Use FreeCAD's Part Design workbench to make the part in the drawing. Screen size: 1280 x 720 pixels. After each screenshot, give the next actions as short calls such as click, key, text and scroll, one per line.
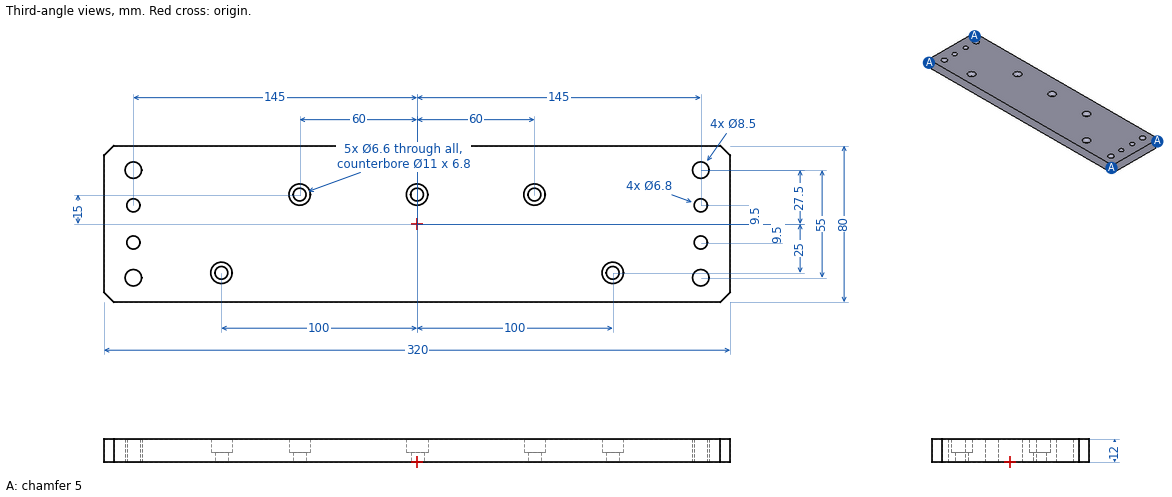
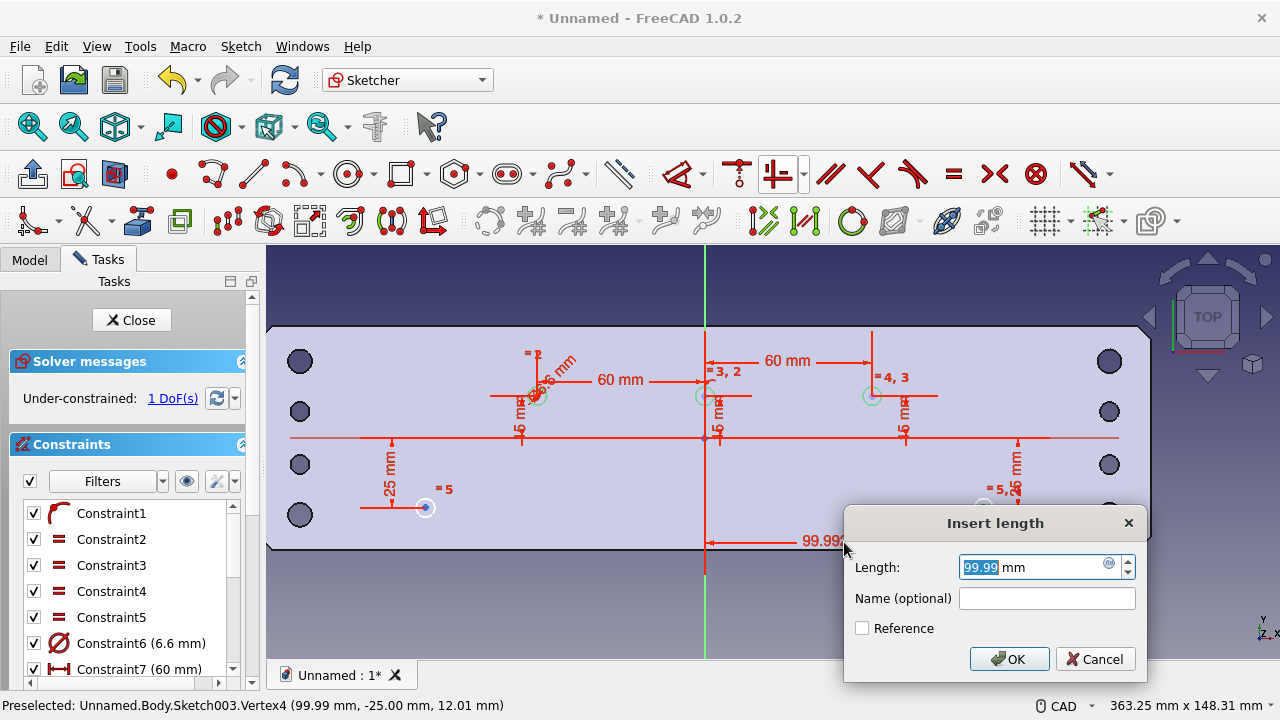
text(100)
key(Return)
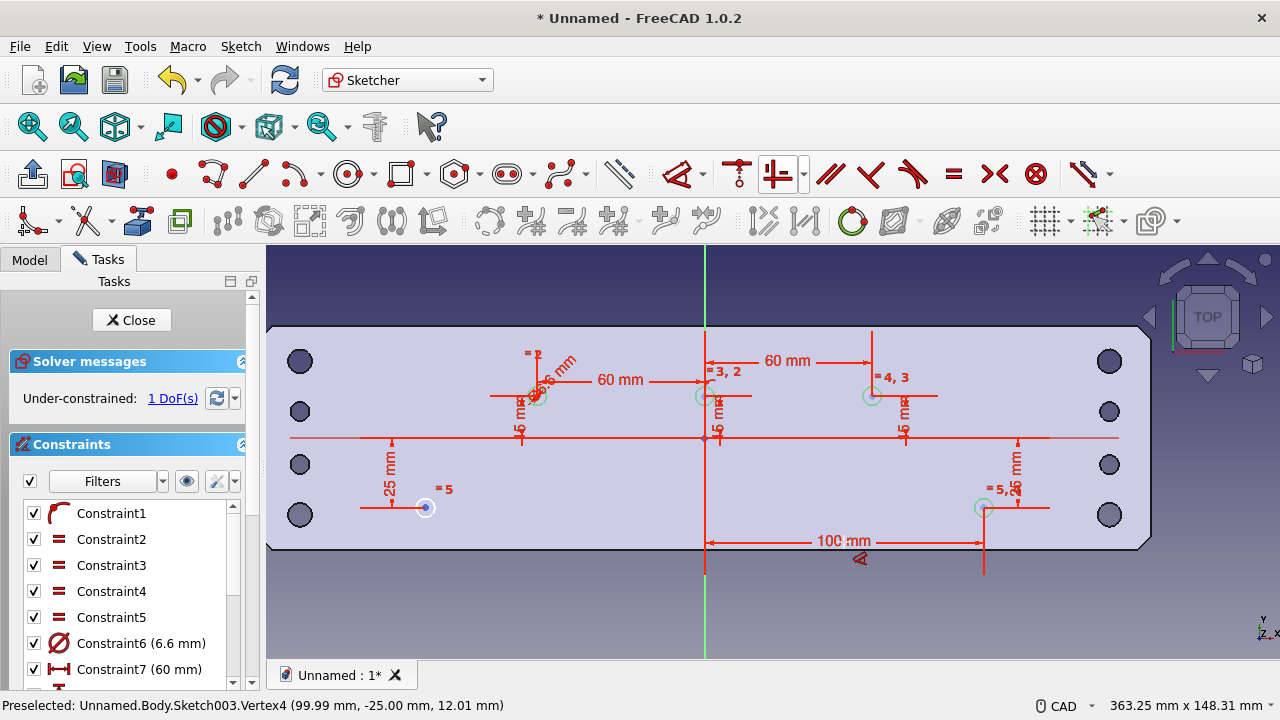
click(426, 508)
click(565, 542)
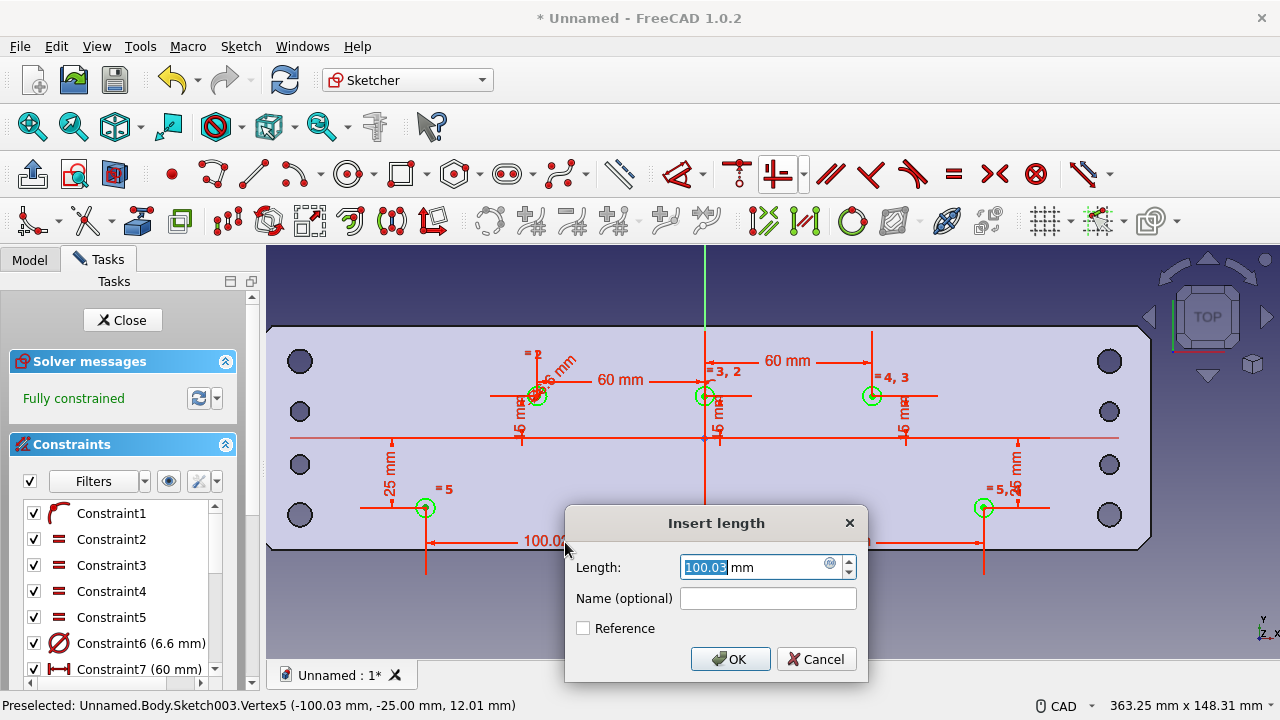
text(100)
key(Return)
key(Escape)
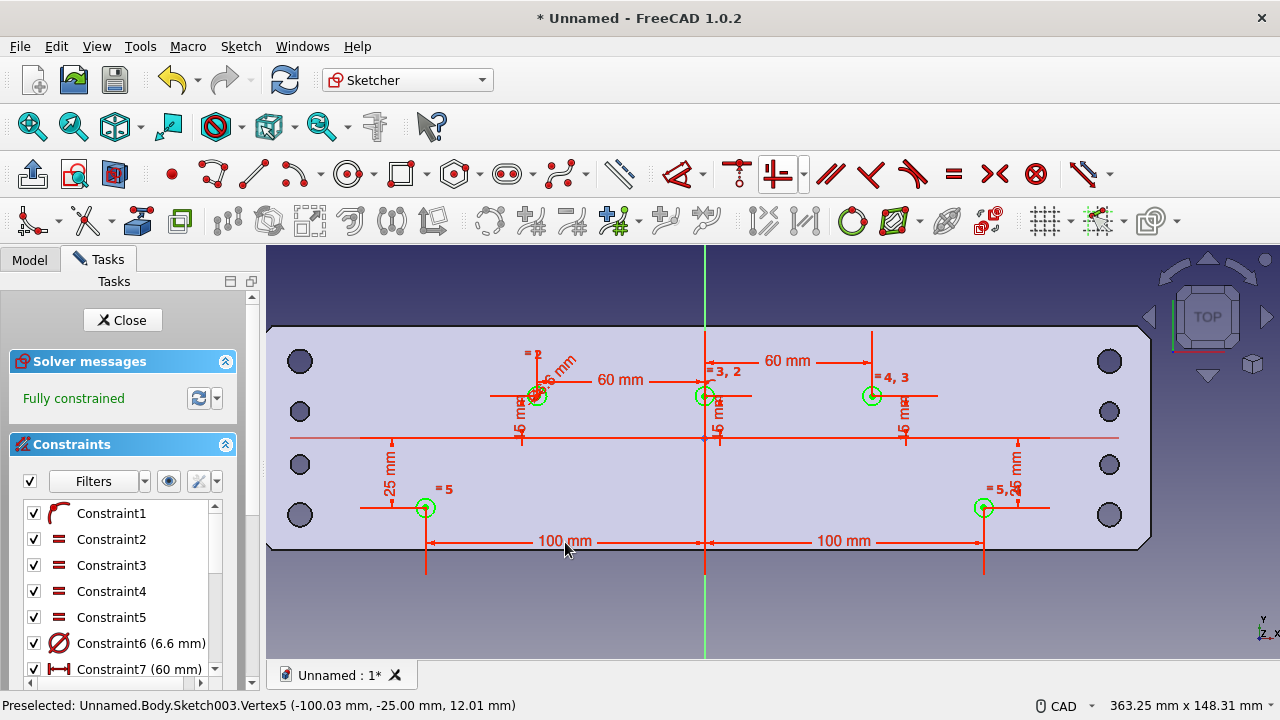
click(123, 320)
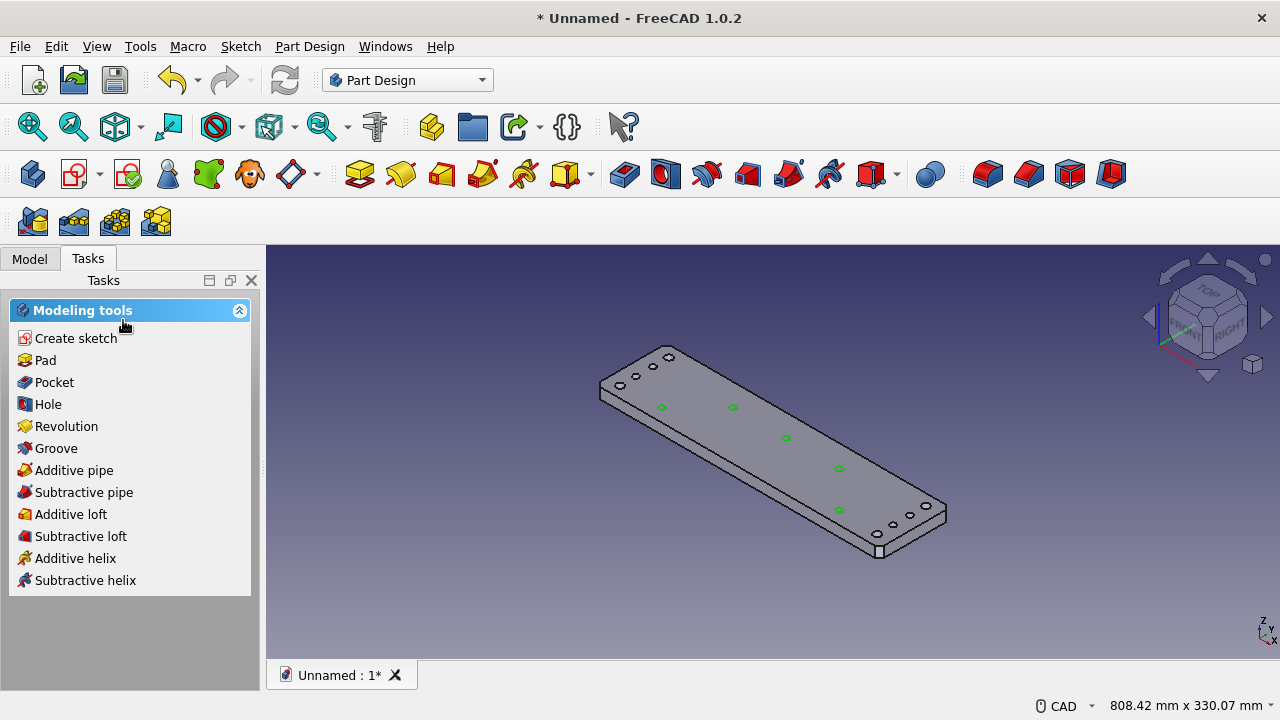
click(666, 174)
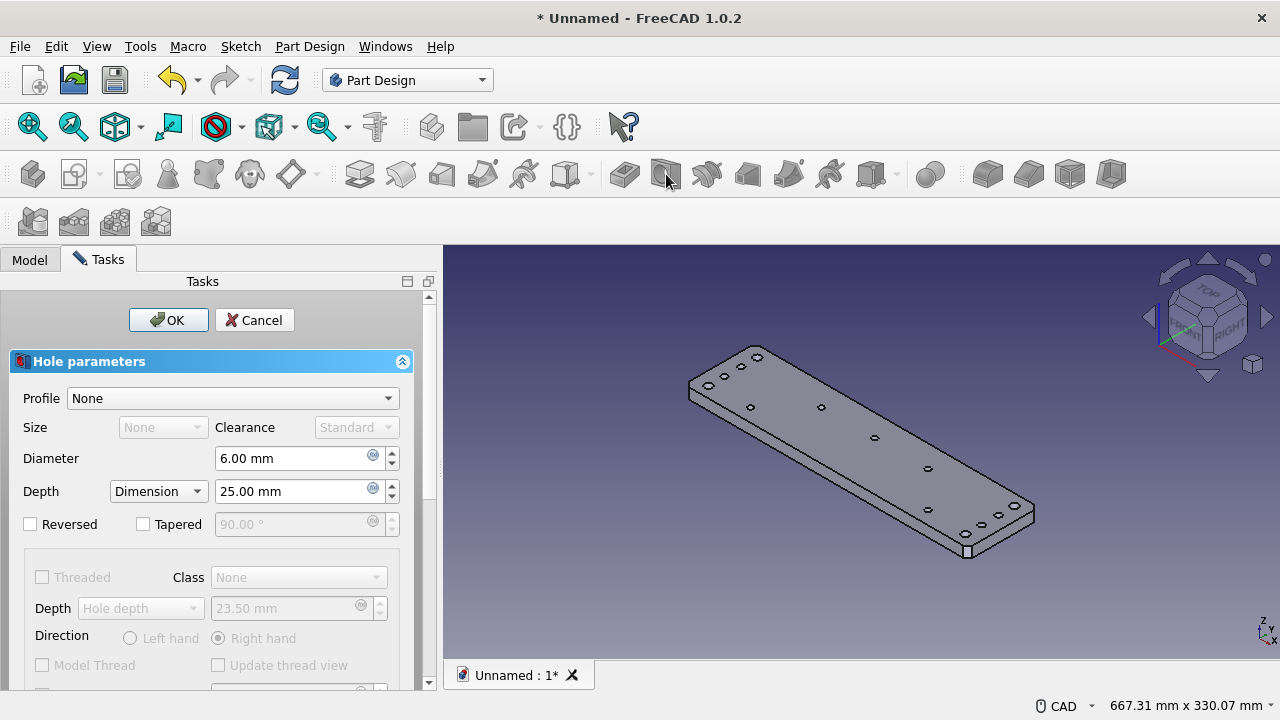
triple_click(300, 458)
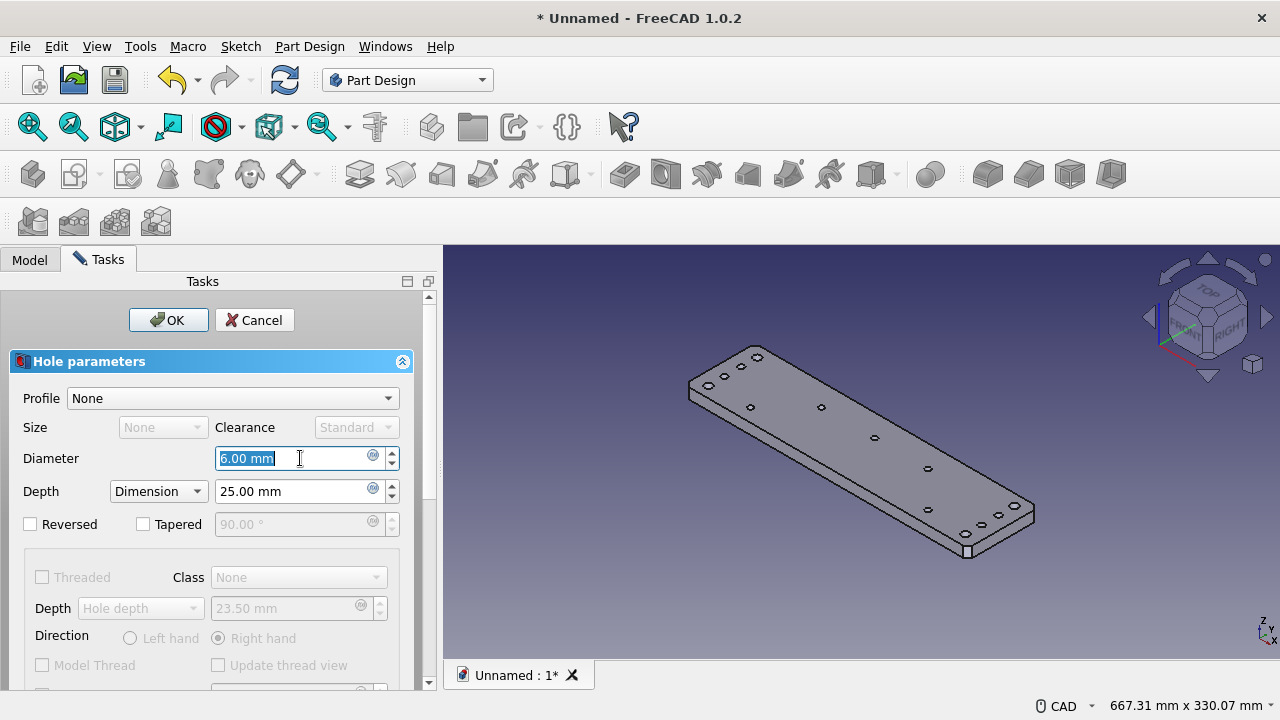
text(6.6)
key(Tab)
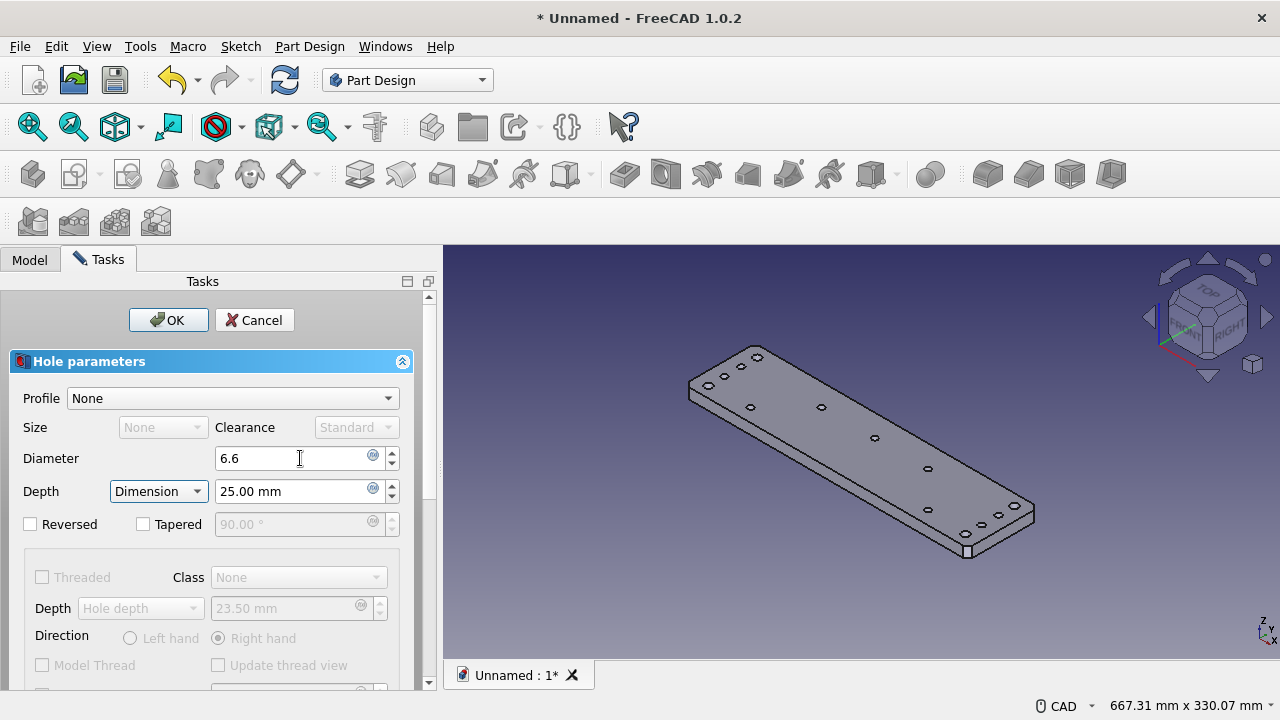
click(160, 492)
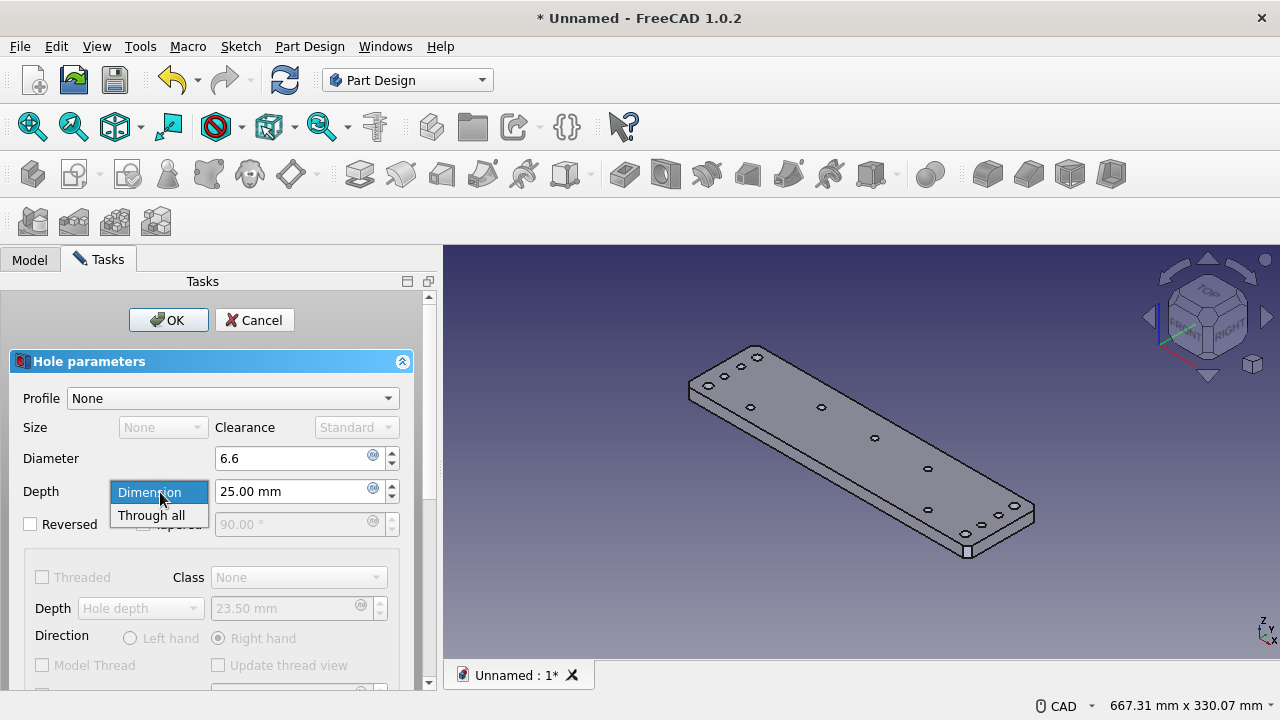
click(158, 516)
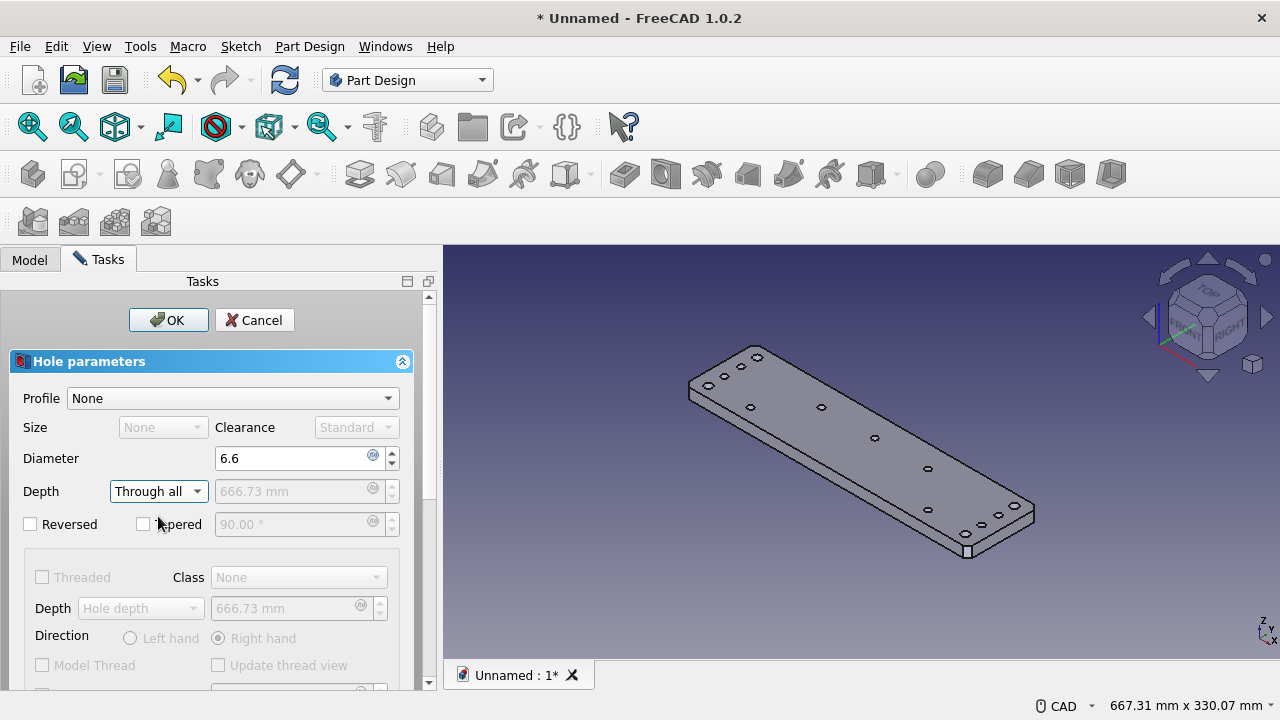
scroll(429, 490, down, 3)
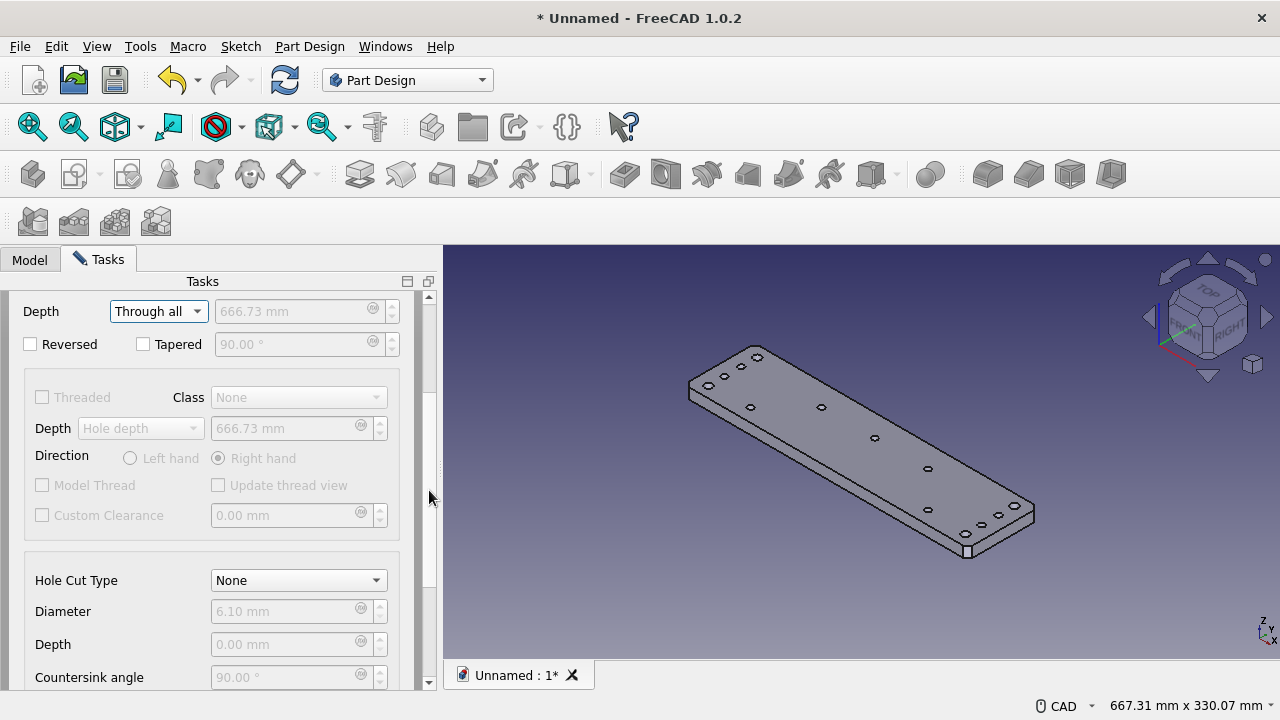
click(300, 580)